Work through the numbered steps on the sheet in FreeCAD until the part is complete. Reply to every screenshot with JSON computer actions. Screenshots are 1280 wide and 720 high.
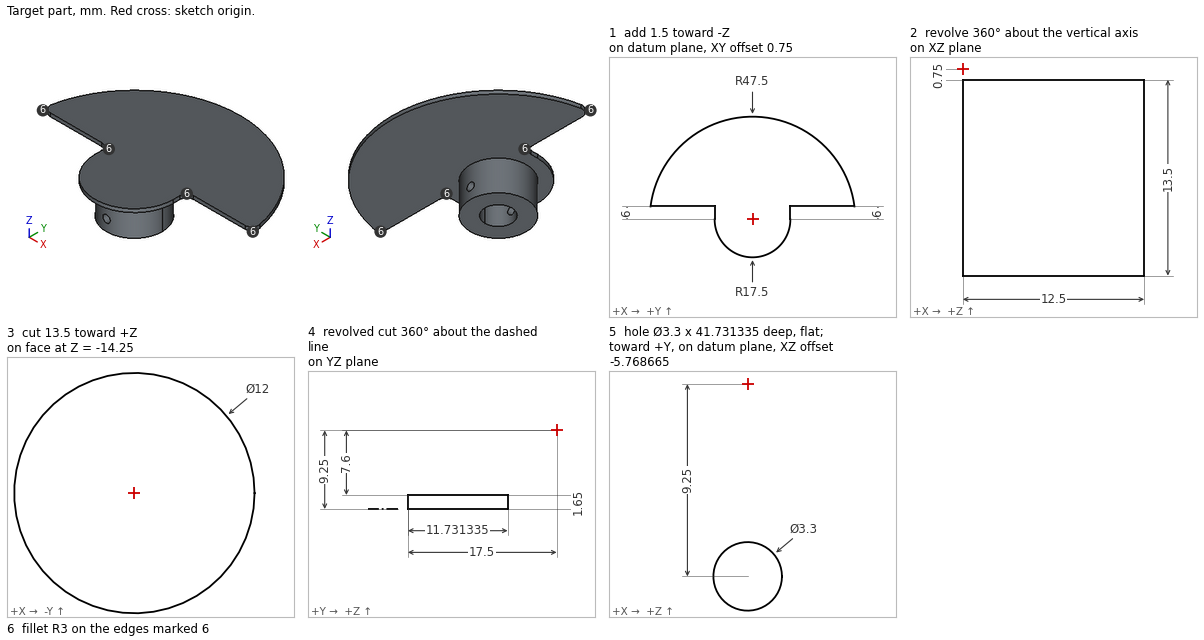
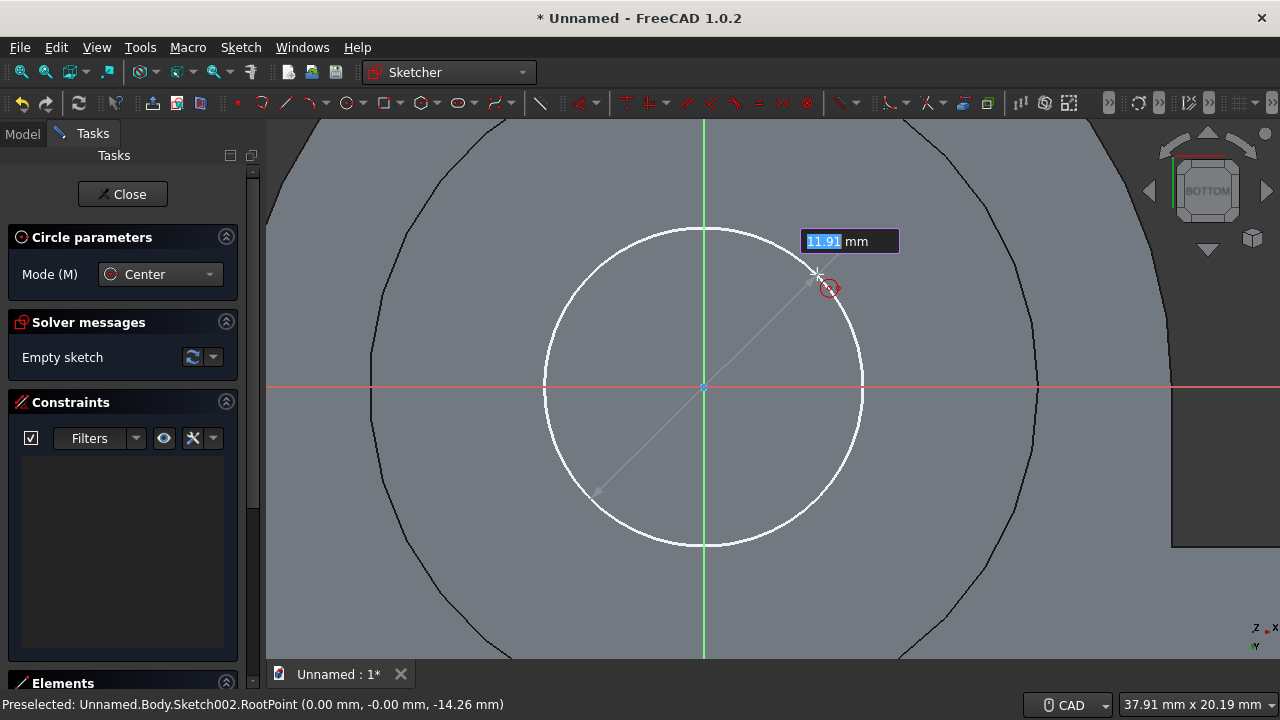
{"action": "type", "text": "12"}
{"action": "key", "text": "Return"}
{"action": "key", "text": "Escape"}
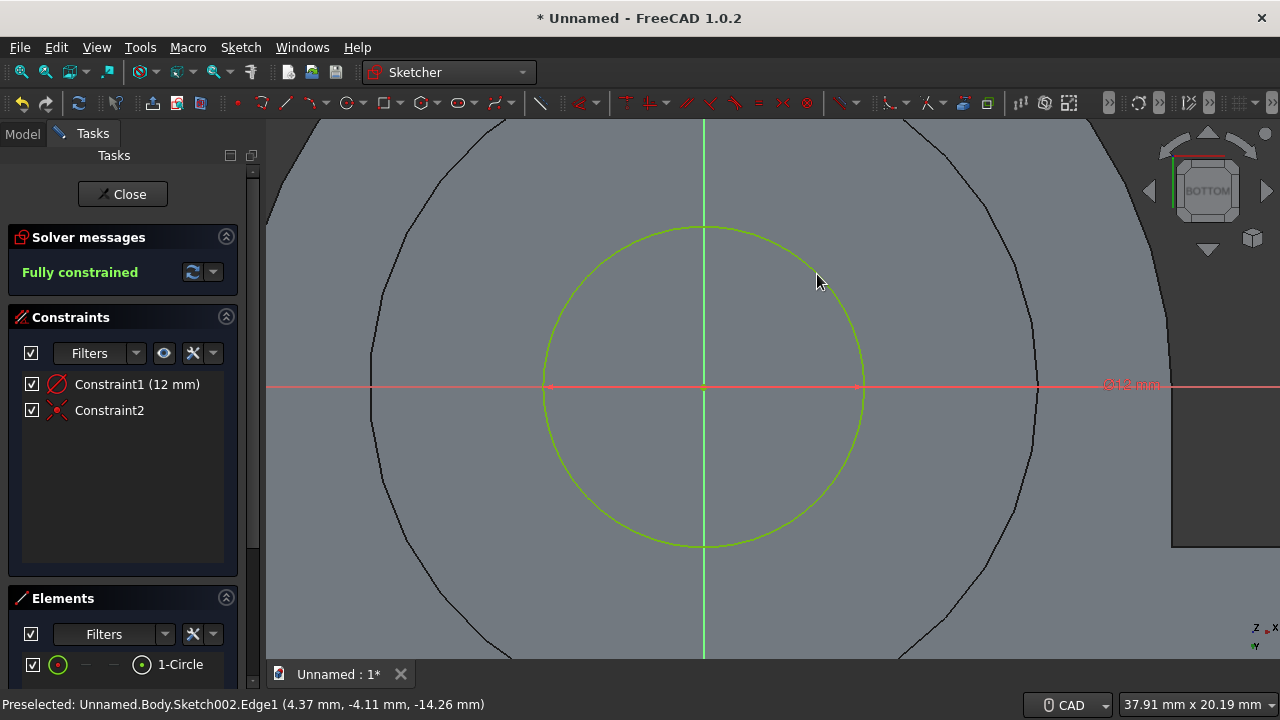
{"action": "left_click", "coordinate": [123, 194]}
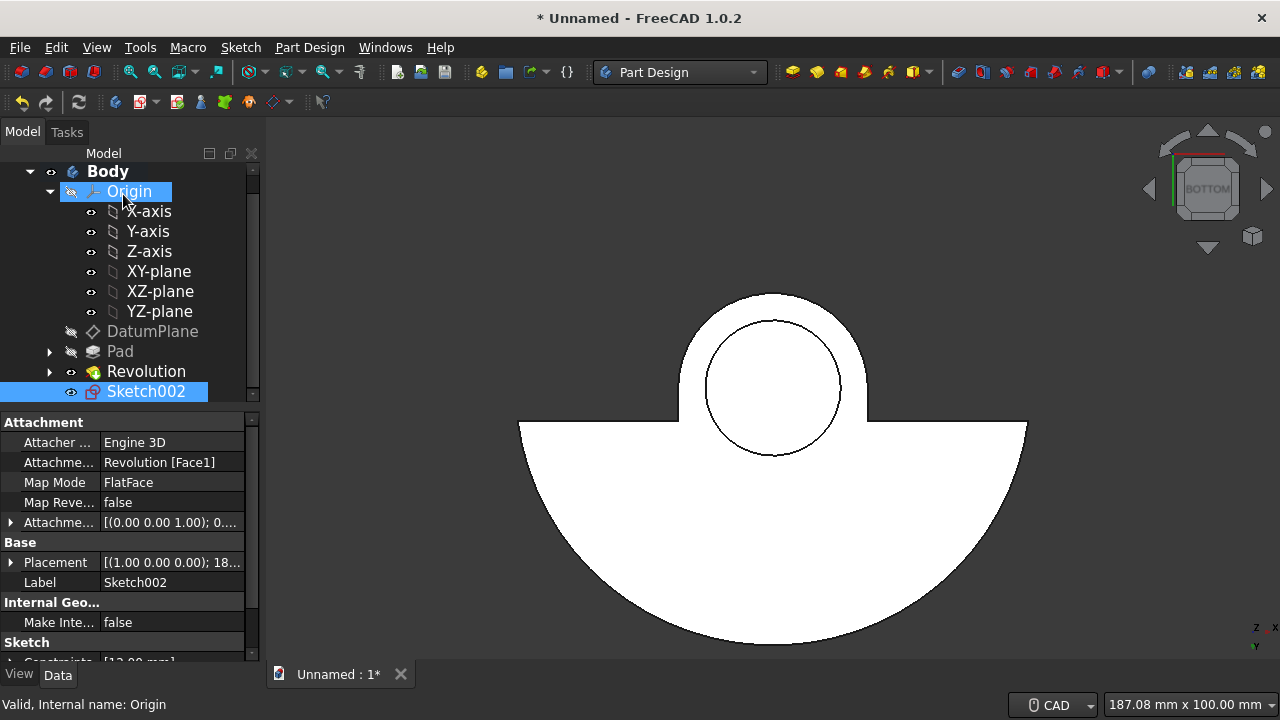
{"action": "left_click", "coordinate": [960, 72]}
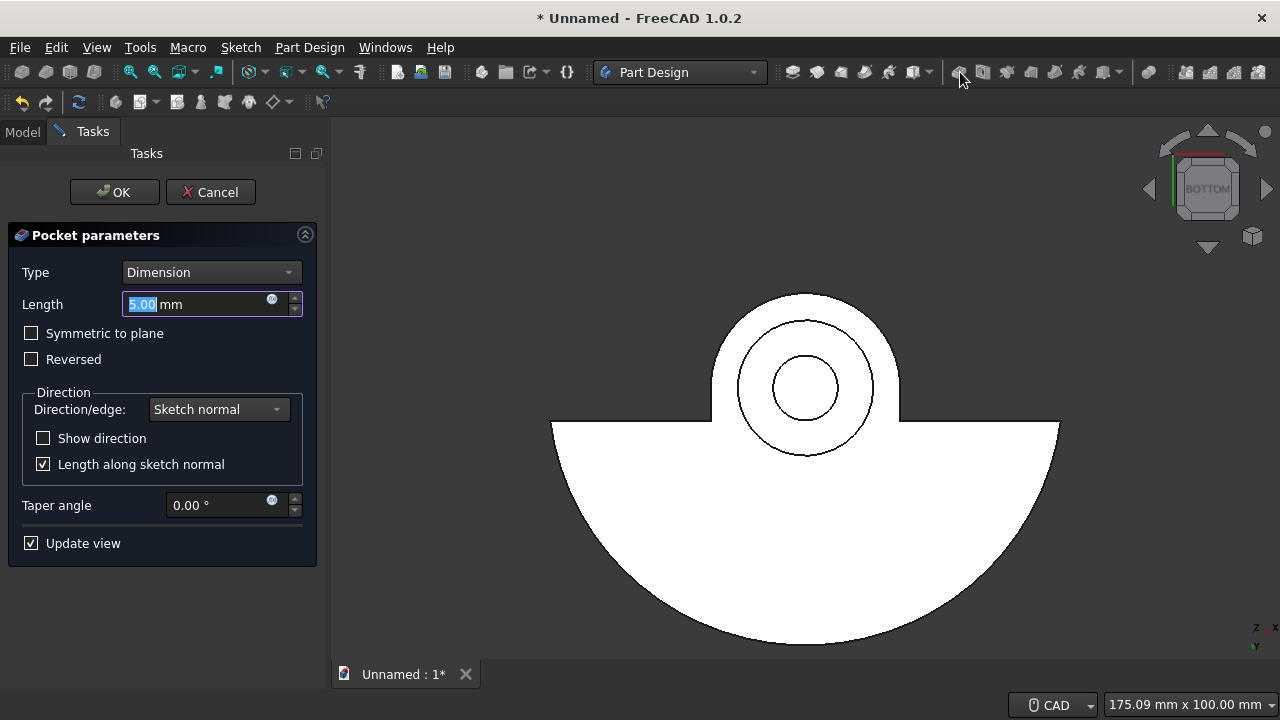
{"action": "type", "text": "13.5"}
{"action": "key", "text": "Tab"}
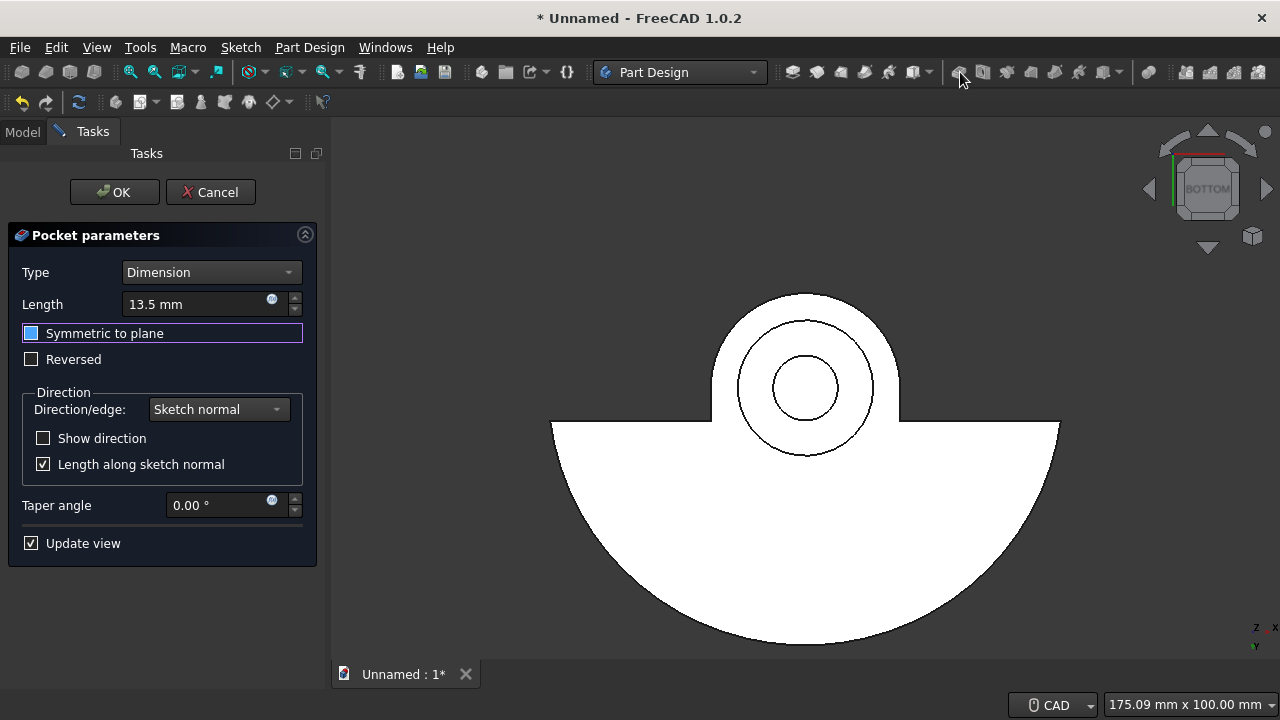
{"action": "left_click", "coordinate": [115, 192]}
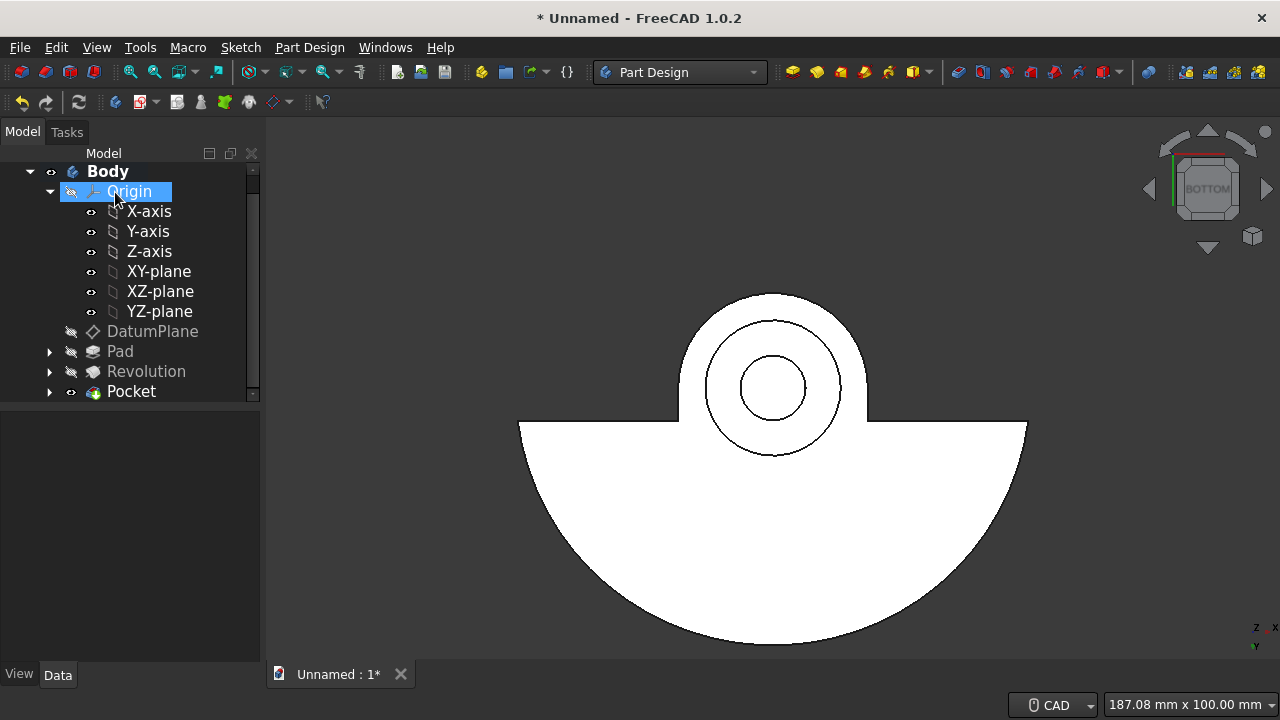
{"action": "left_click", "coordinate": [140, 102]}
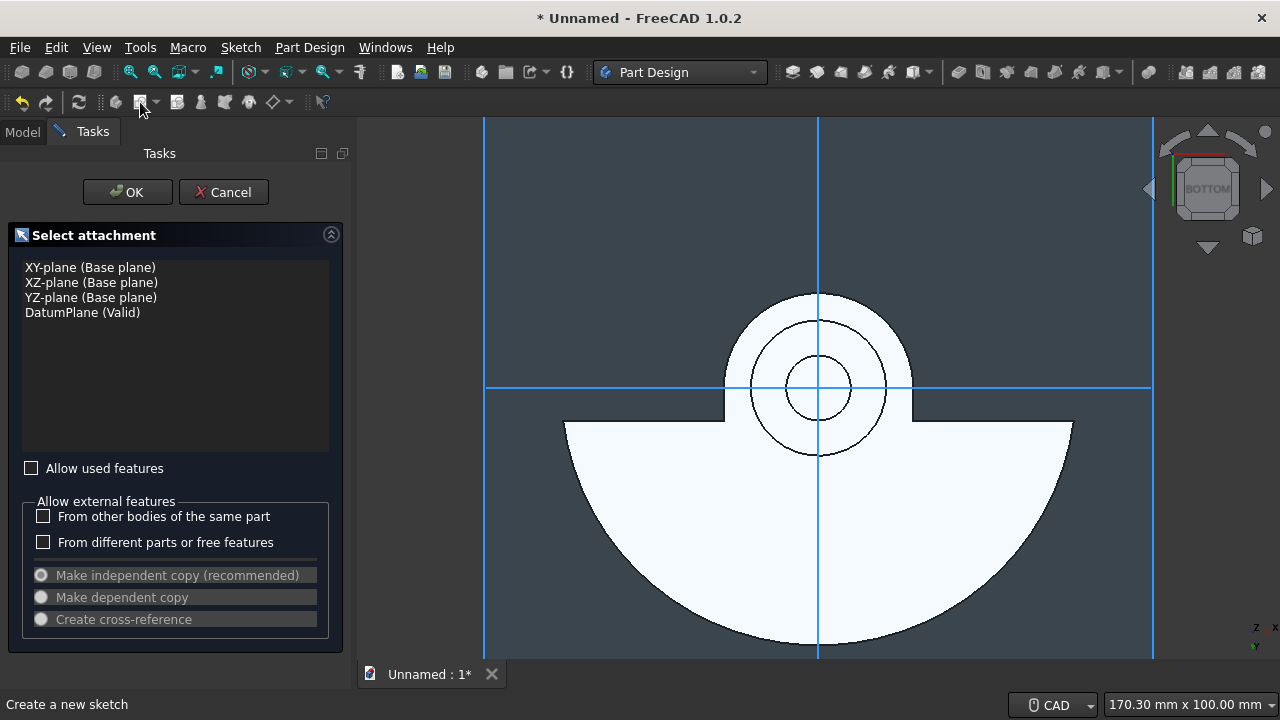
{"action": "left_click", "coordinate": [82, 298]}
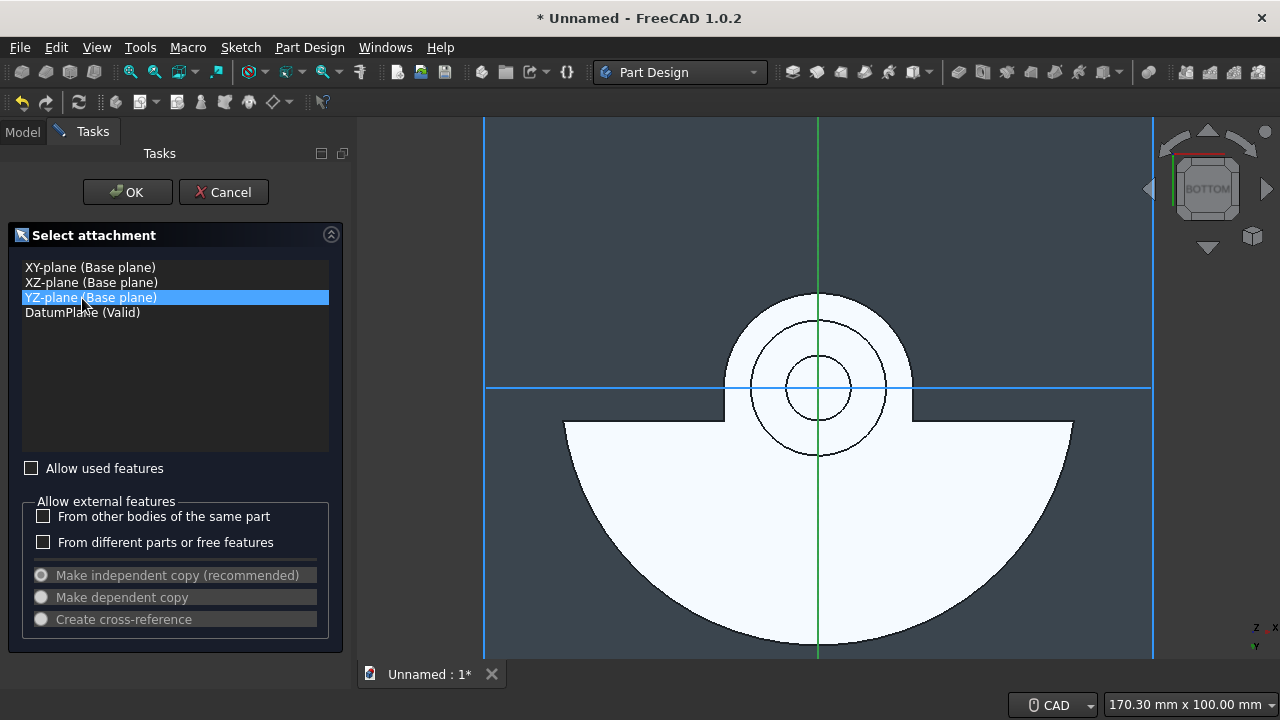
{"action": "left_click", "coordinate": [128, 192]}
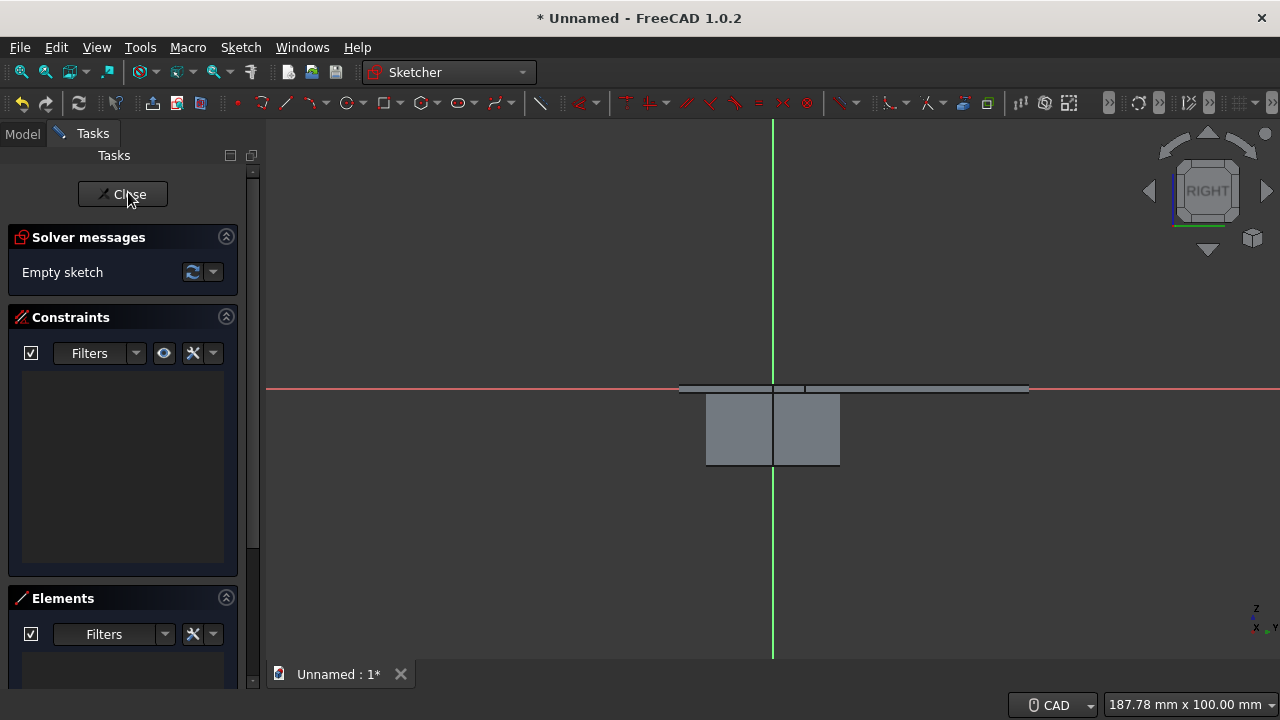
{"action": "key", "text": "q s"}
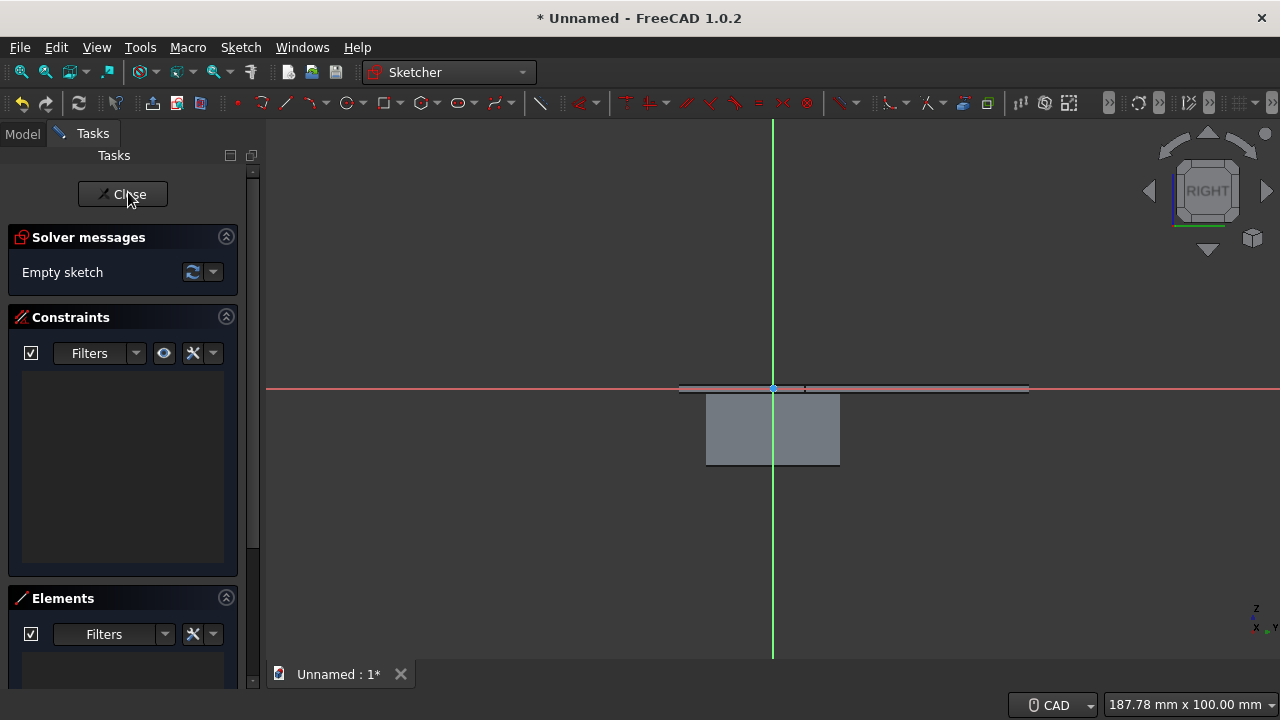
{"action": "scroll", "coordinate": [715, 420], "scroll_direction": "up", "scroll_amount": 8}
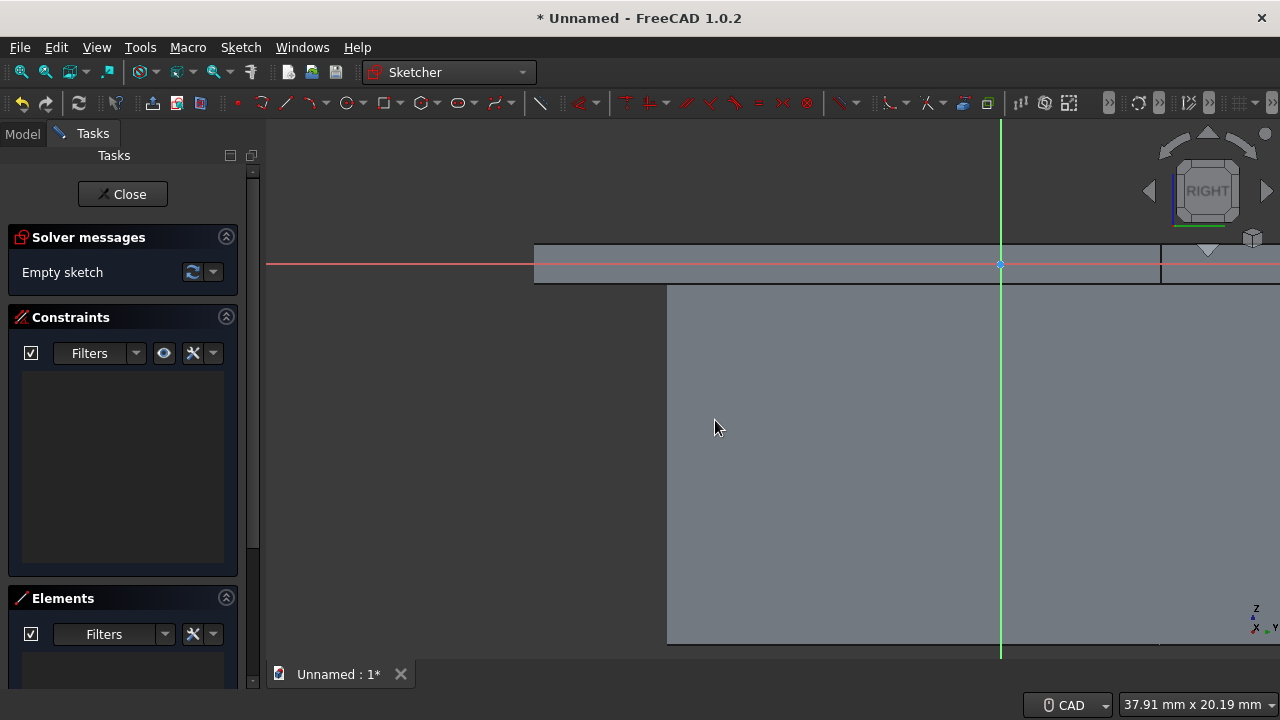
{"action": "left_click", "coordinate": [384, 104]}